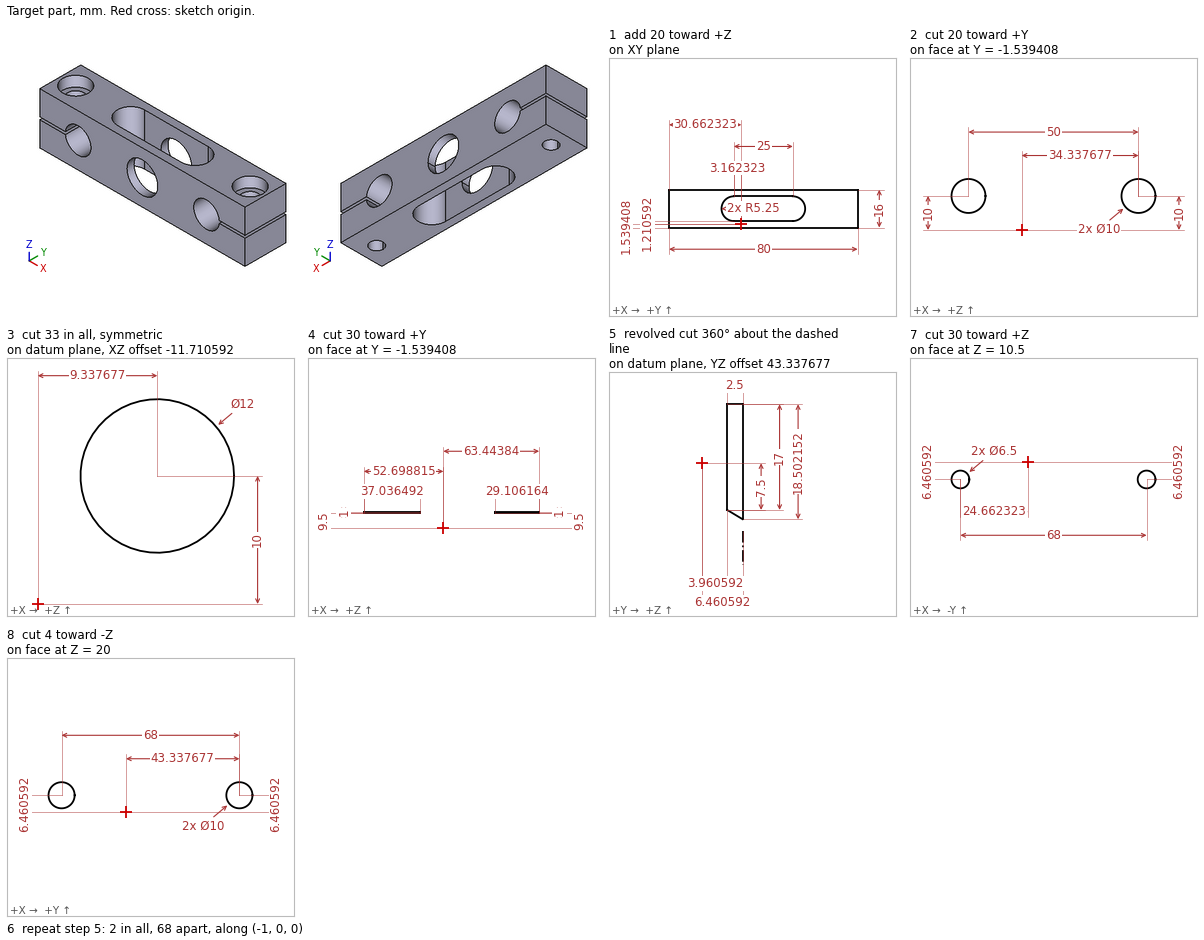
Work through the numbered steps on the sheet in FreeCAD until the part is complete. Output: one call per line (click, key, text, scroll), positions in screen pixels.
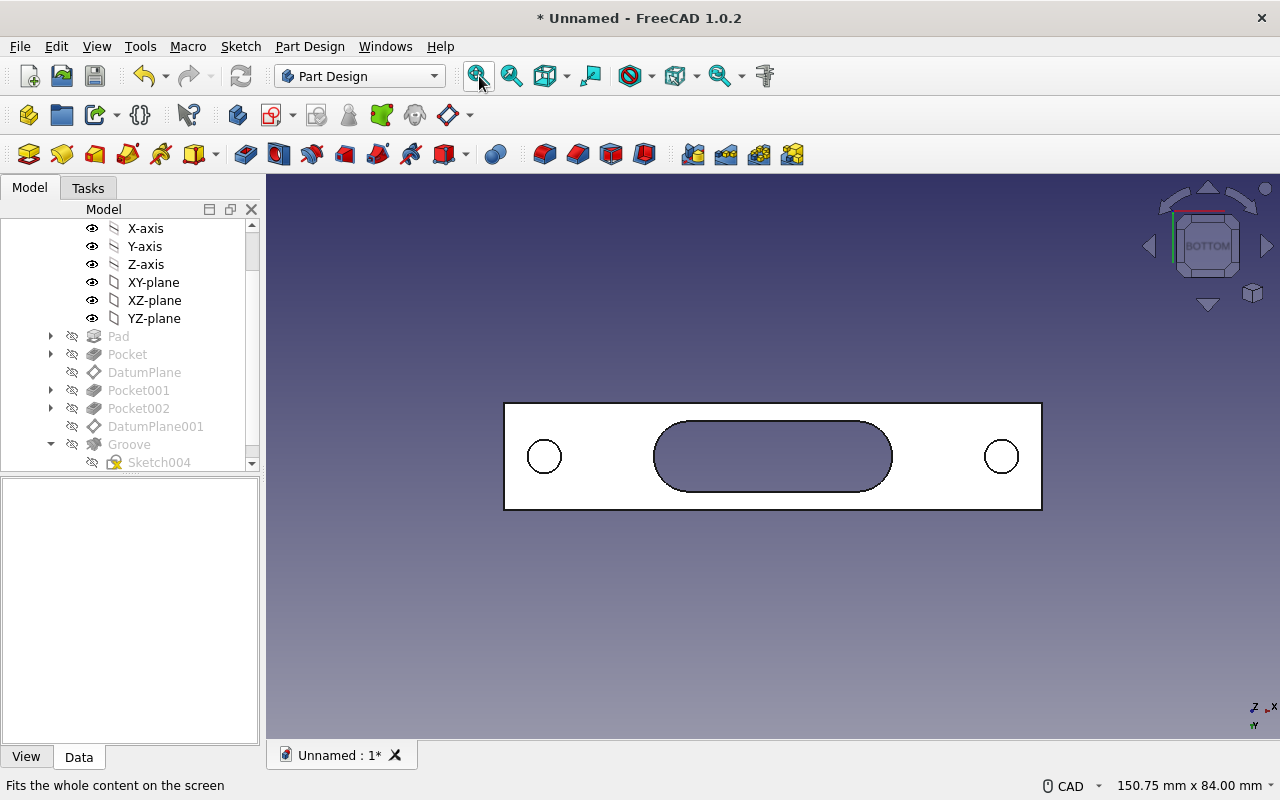
click(1008, 455)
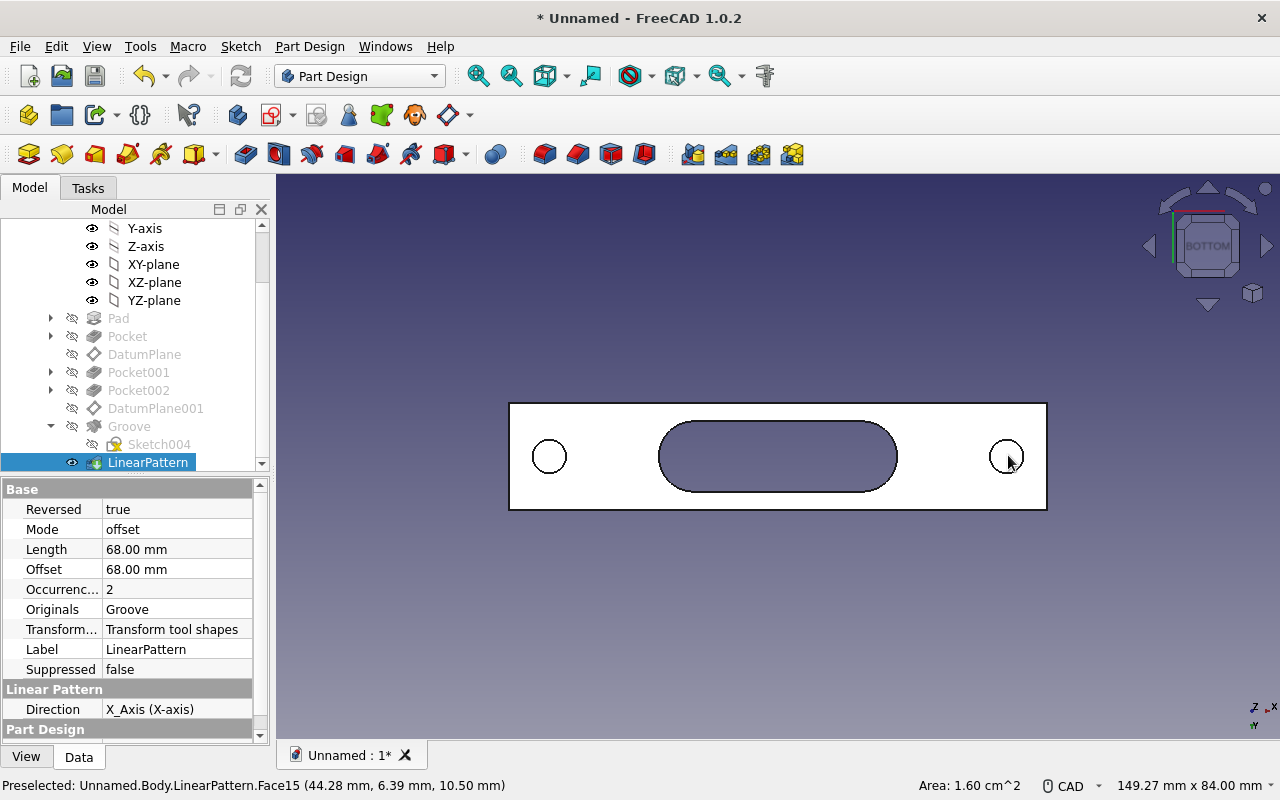
click(270, 116)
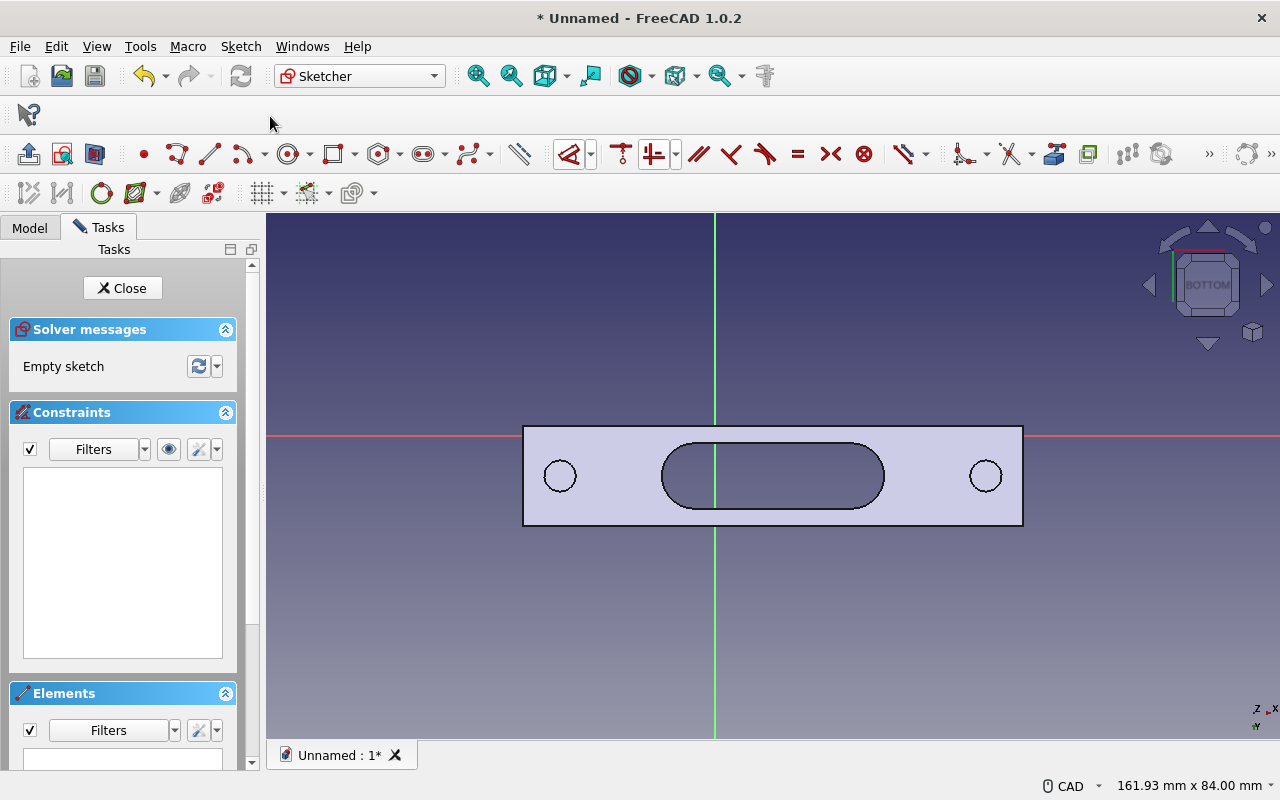
click(288, 154)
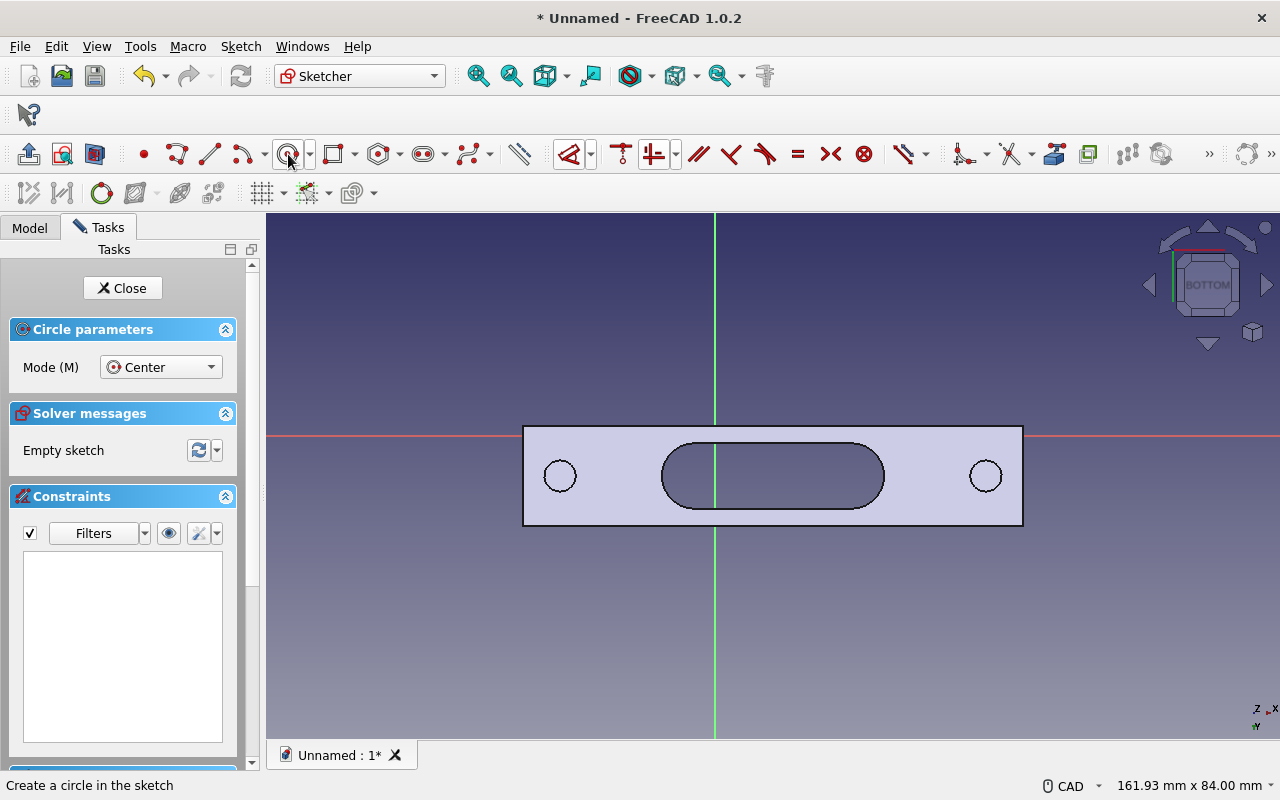
click(560, 476)
move(574, 462)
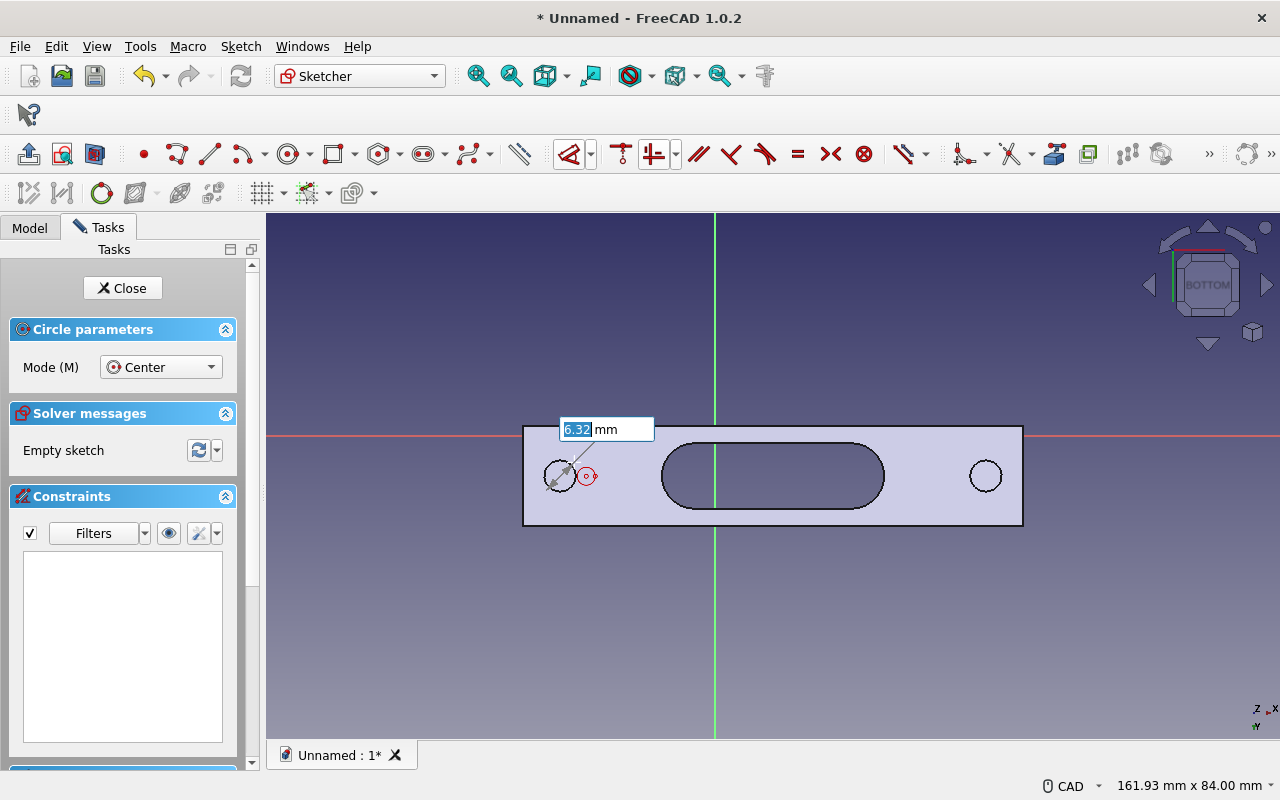
text(6.5)
key(Return)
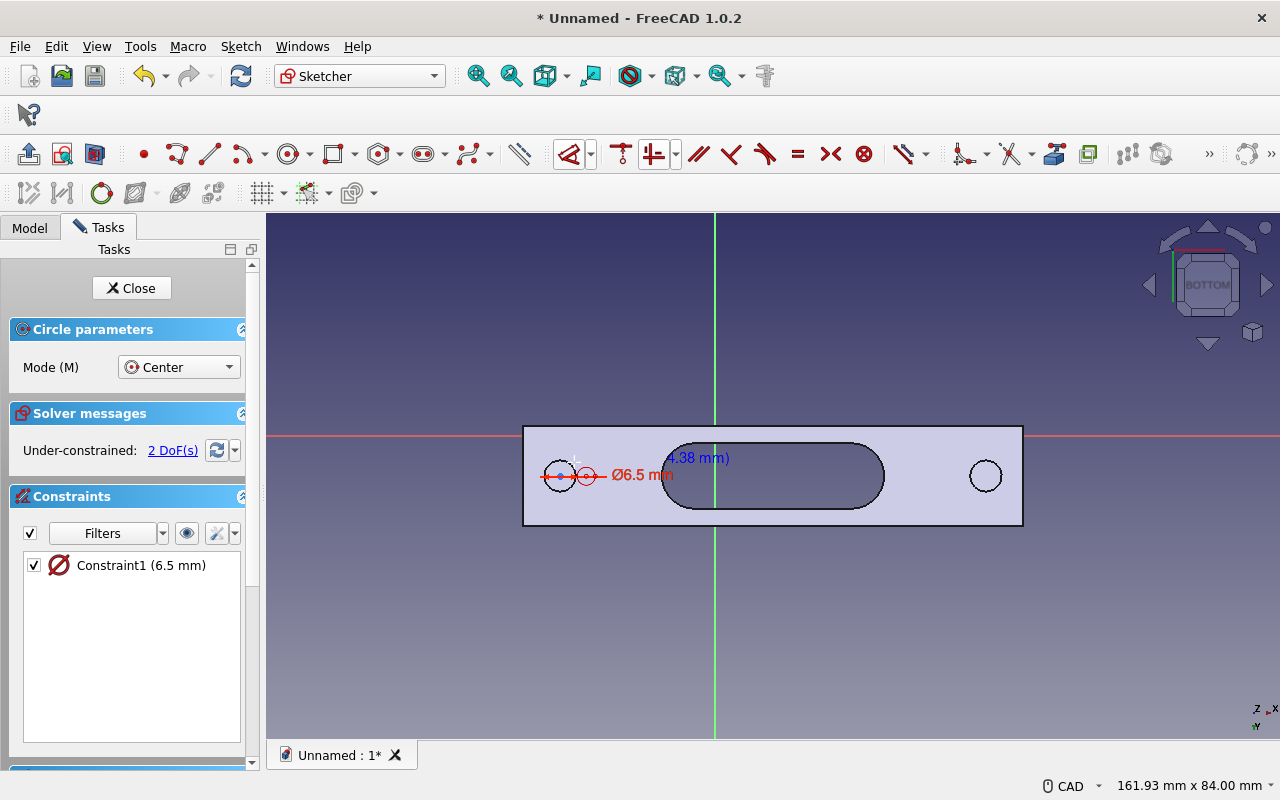
click(986, 476)
move(1000, 462)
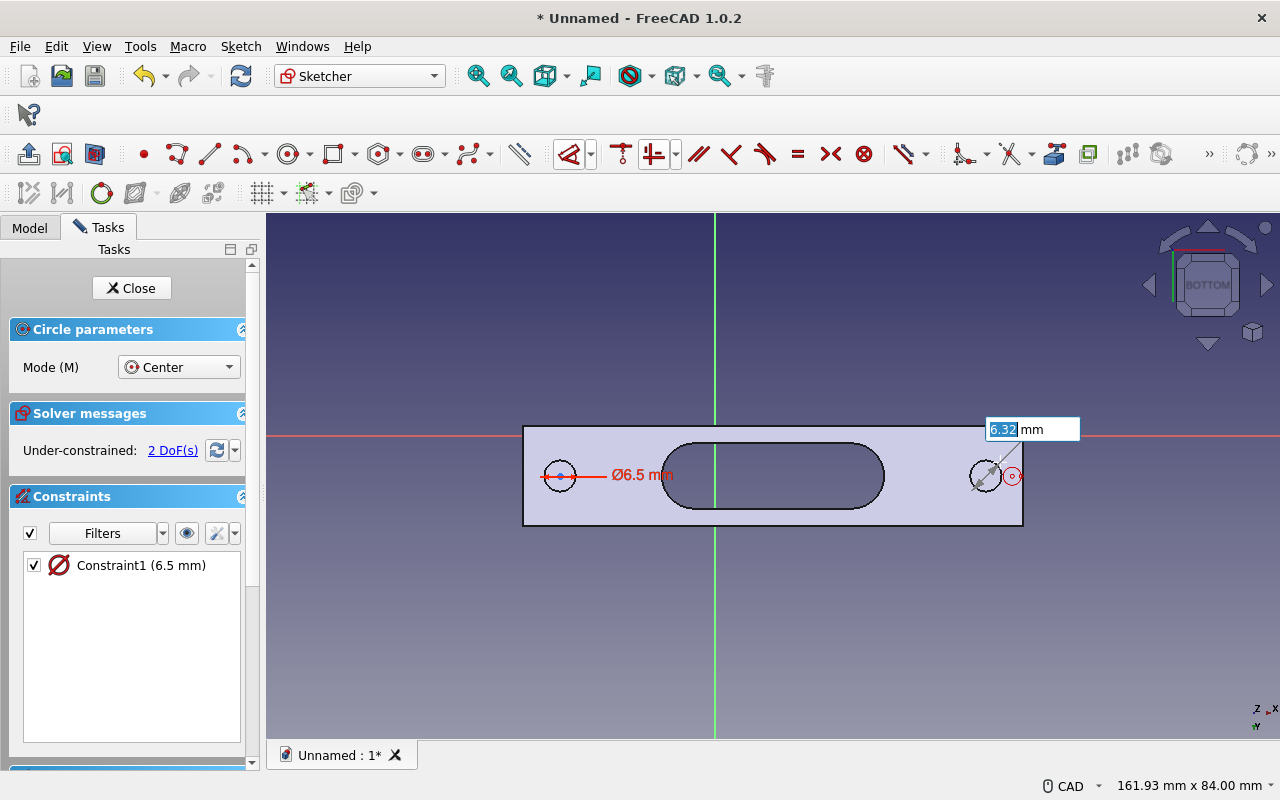
text(6.5)
key(Return)
key(Escape)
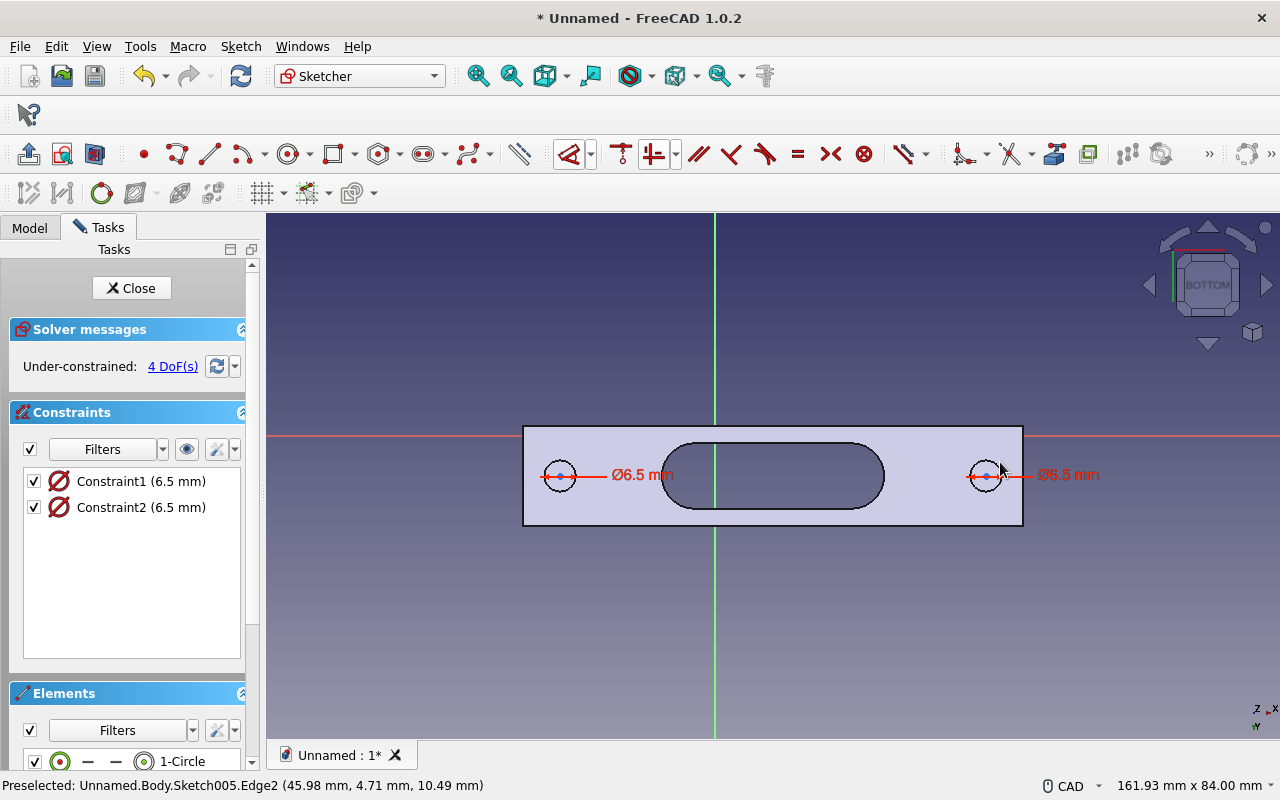
click(560, 477)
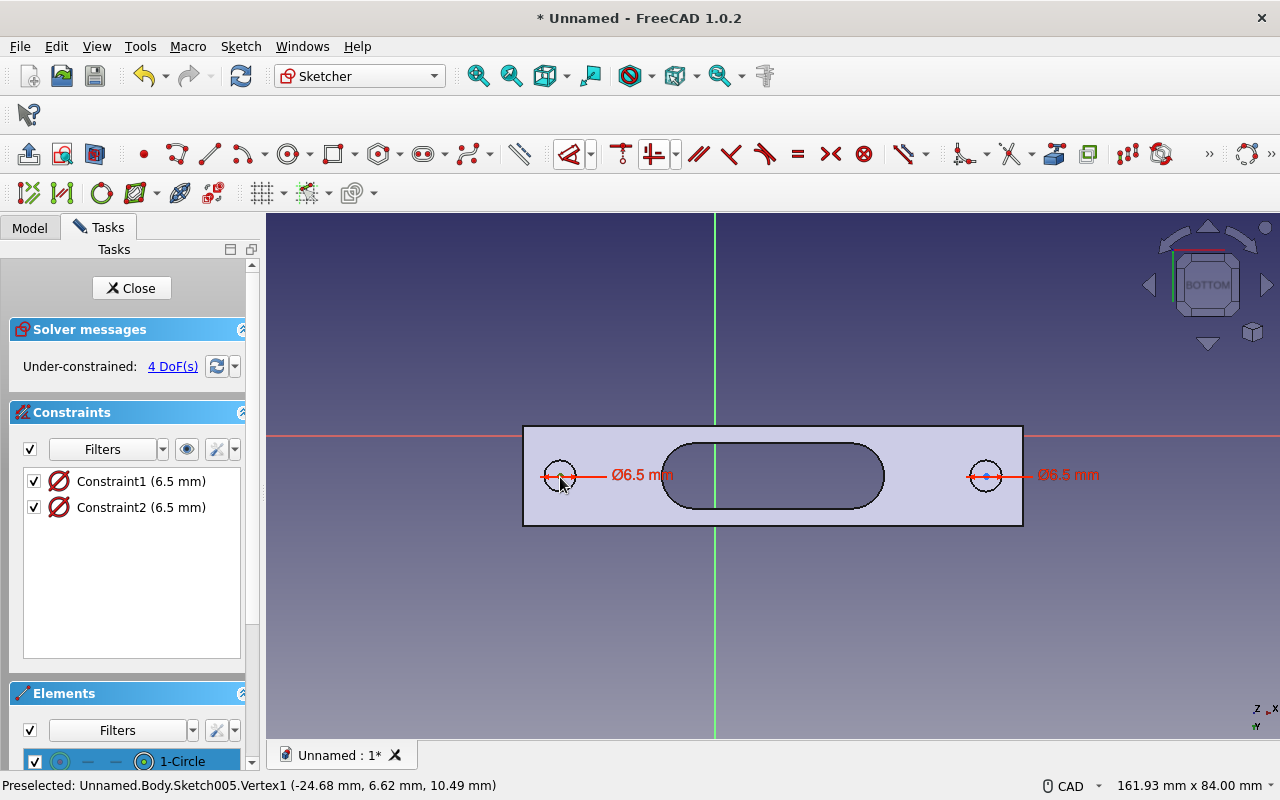
click(986, 477)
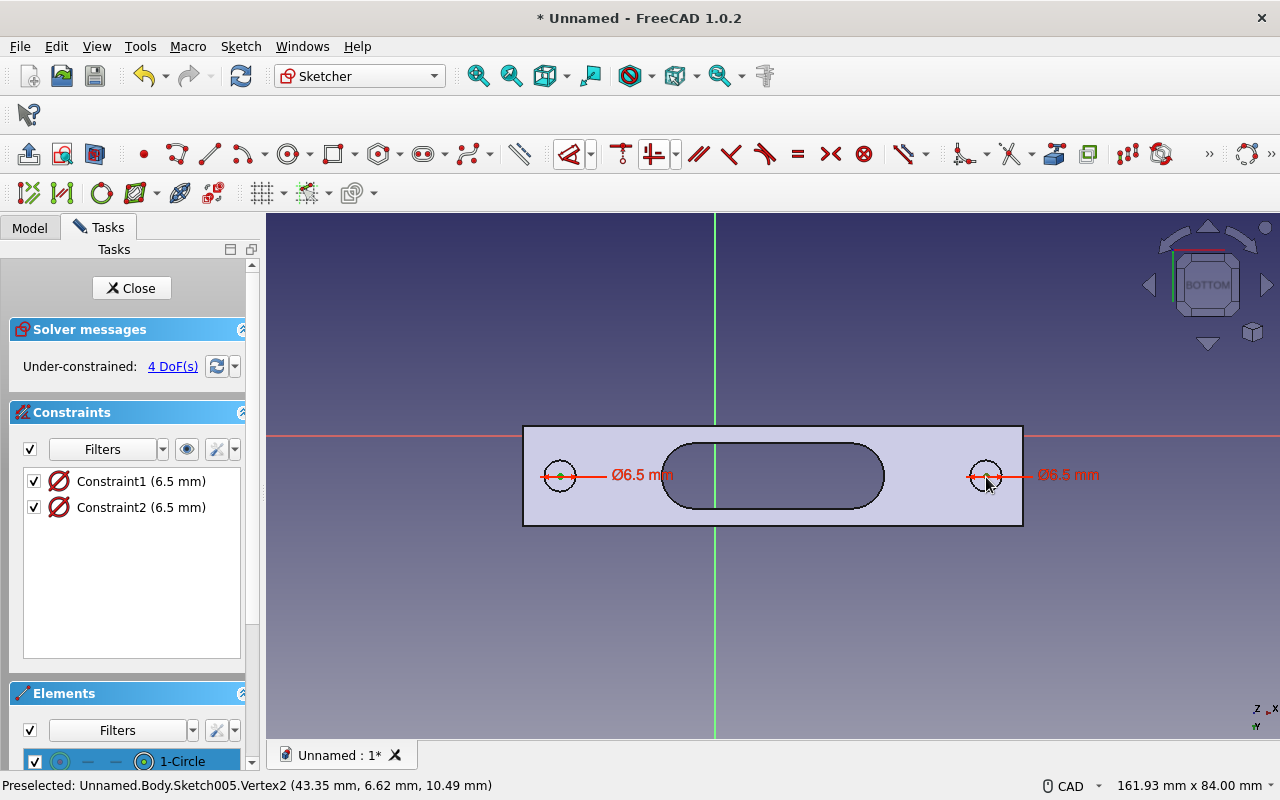
key(l)